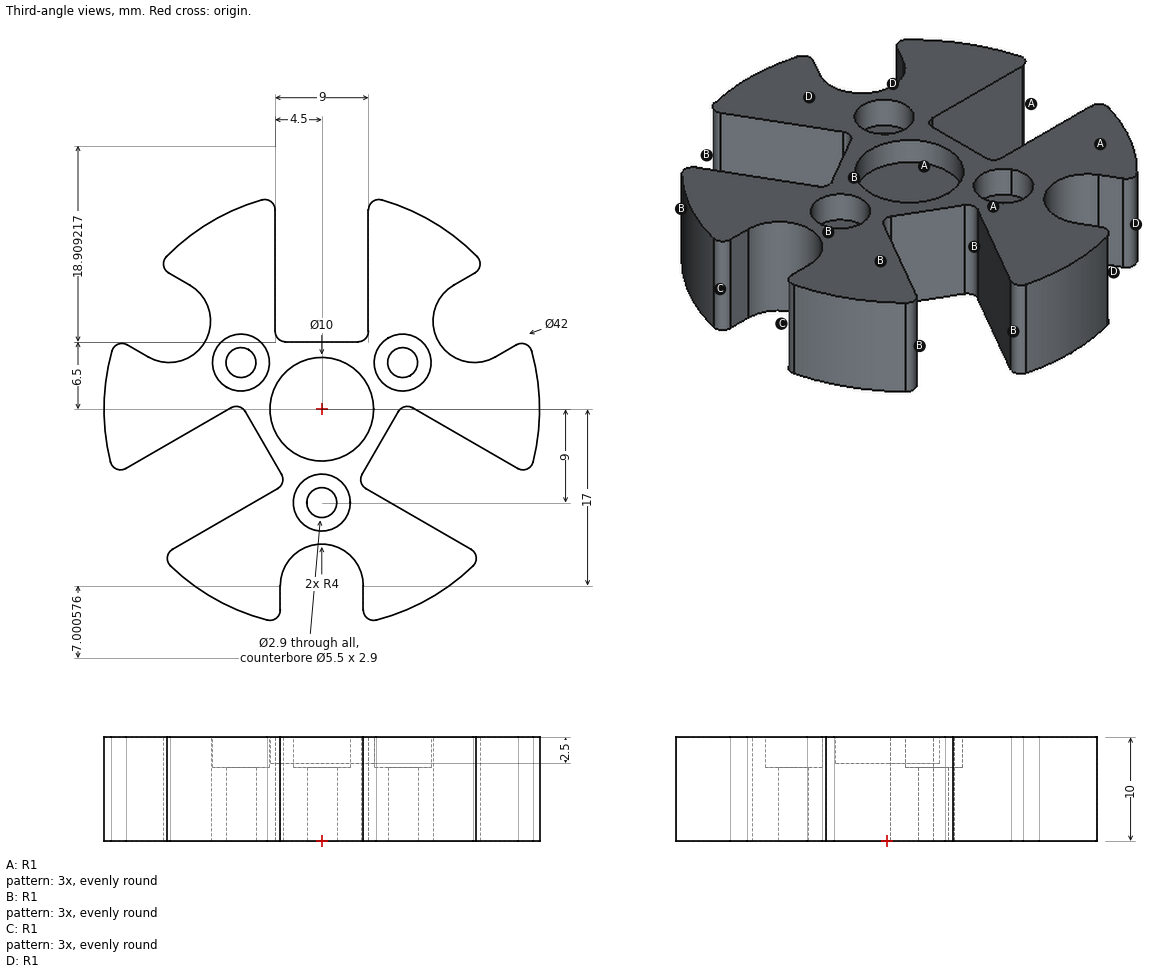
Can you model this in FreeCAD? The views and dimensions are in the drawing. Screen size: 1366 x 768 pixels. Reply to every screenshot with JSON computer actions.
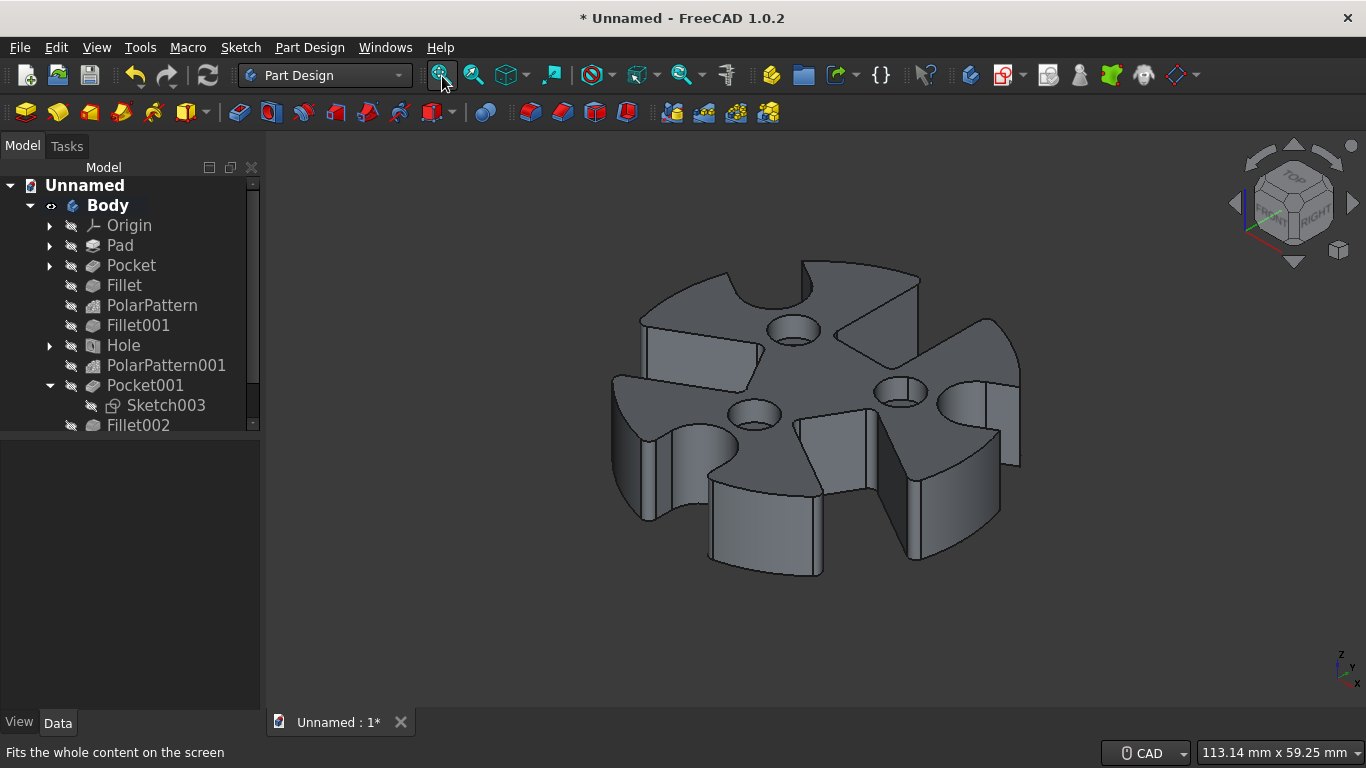
{"action": "left_click", "coordinate": [1020, 426]}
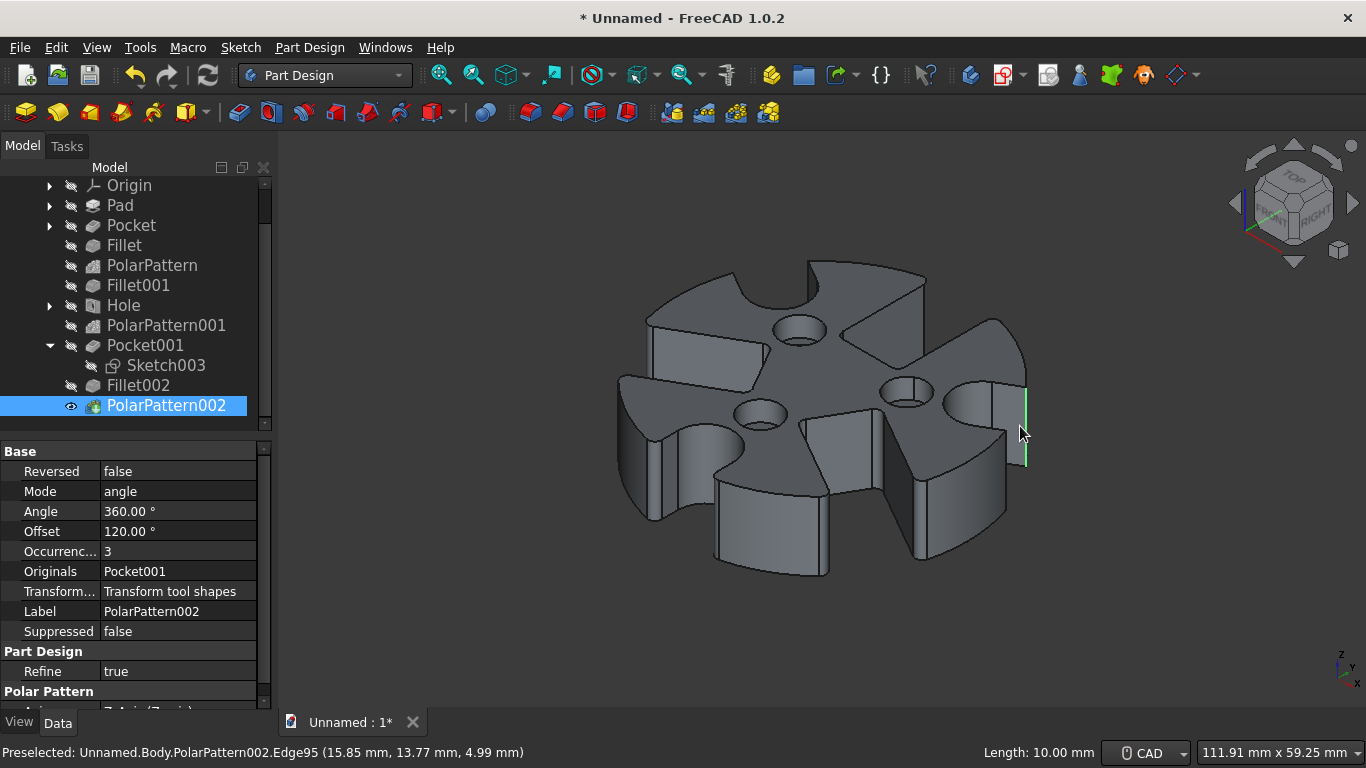
{"action": "key", "text": "2"}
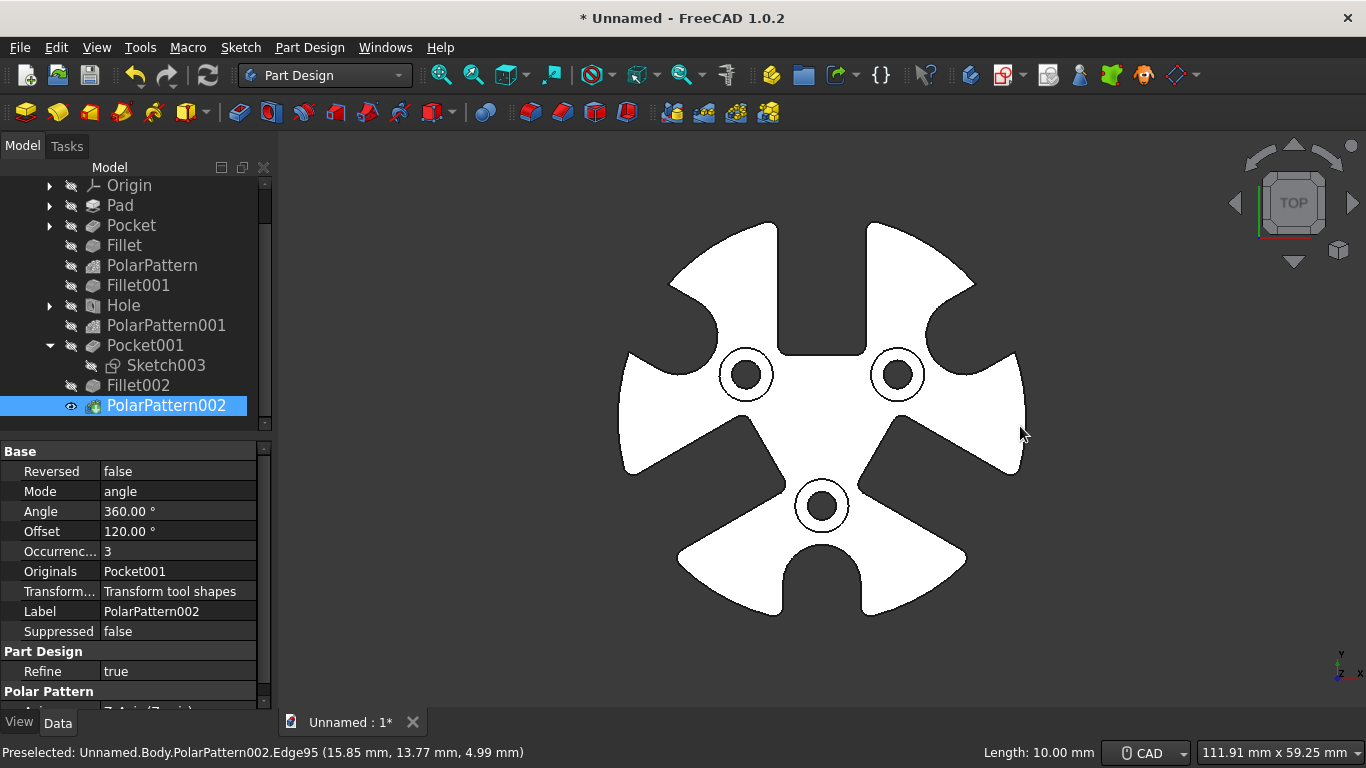
{"action": "key", "text": "1"}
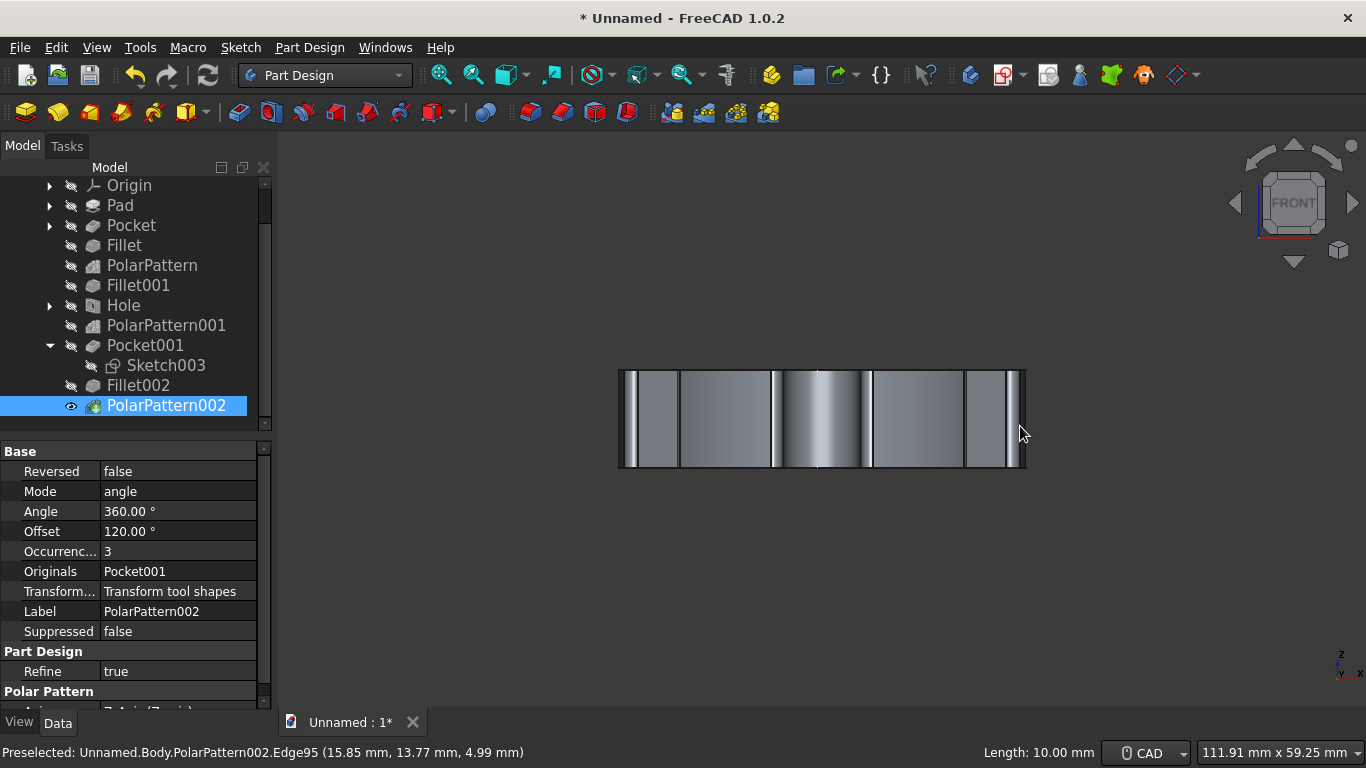
{"action": "left_click", "coordinate": [442, 76]}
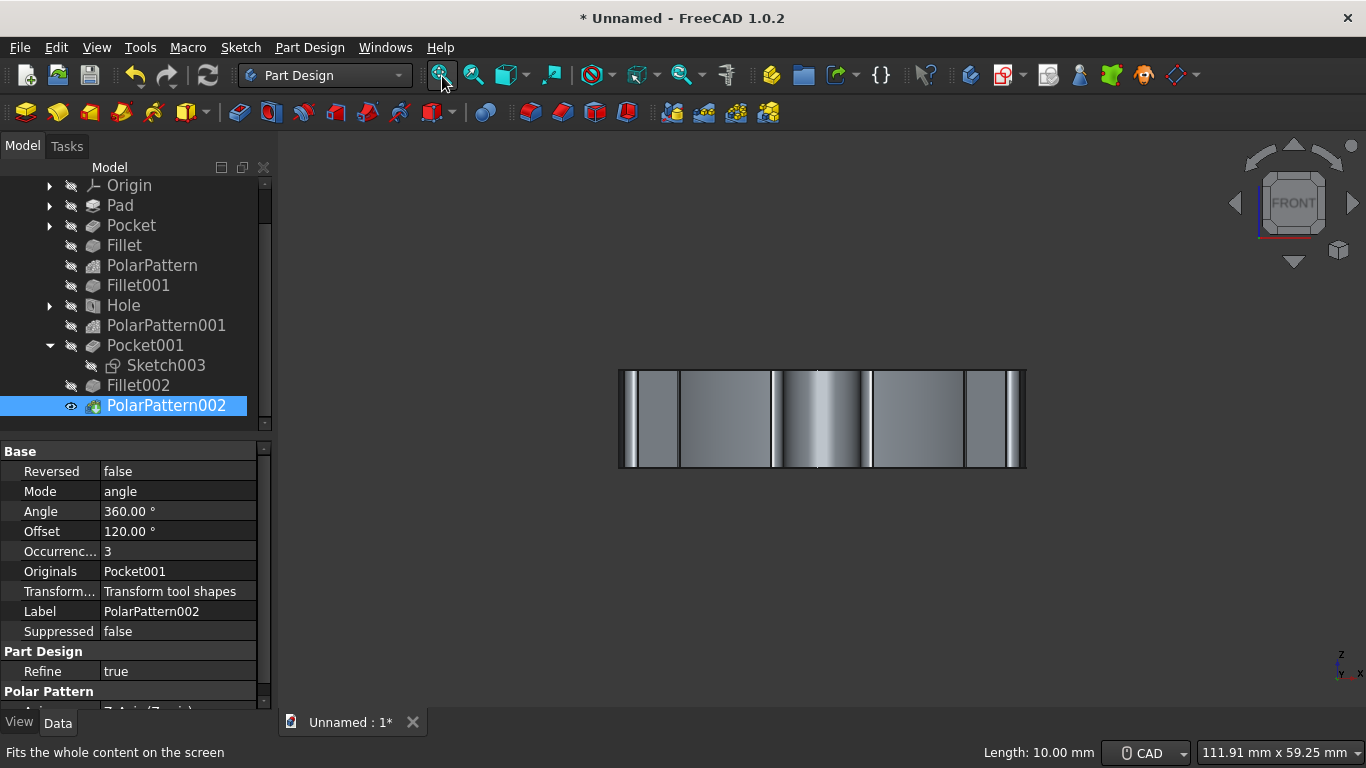
{"action": "key", "text": "3"}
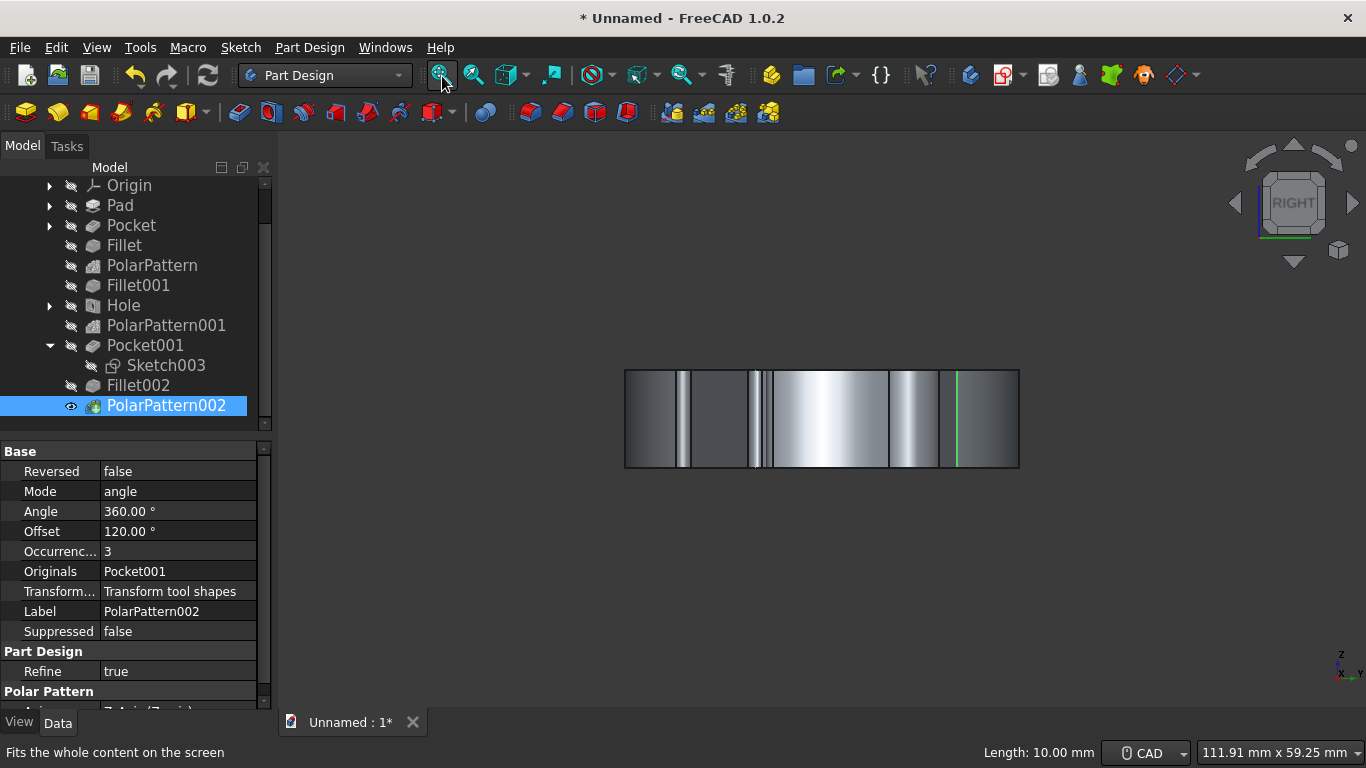
{"action": "left_click", "coordinate": [442, 76]}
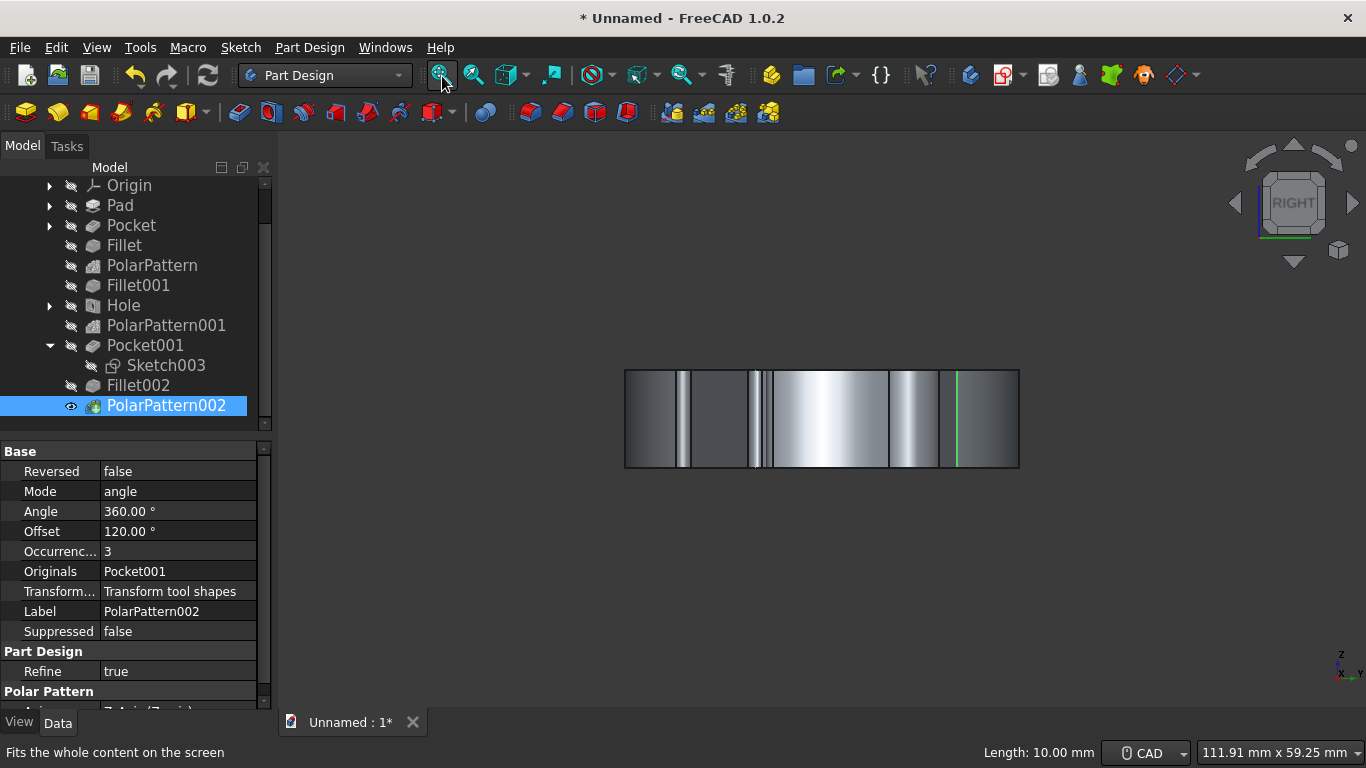
{"action": "key", "text": "5"}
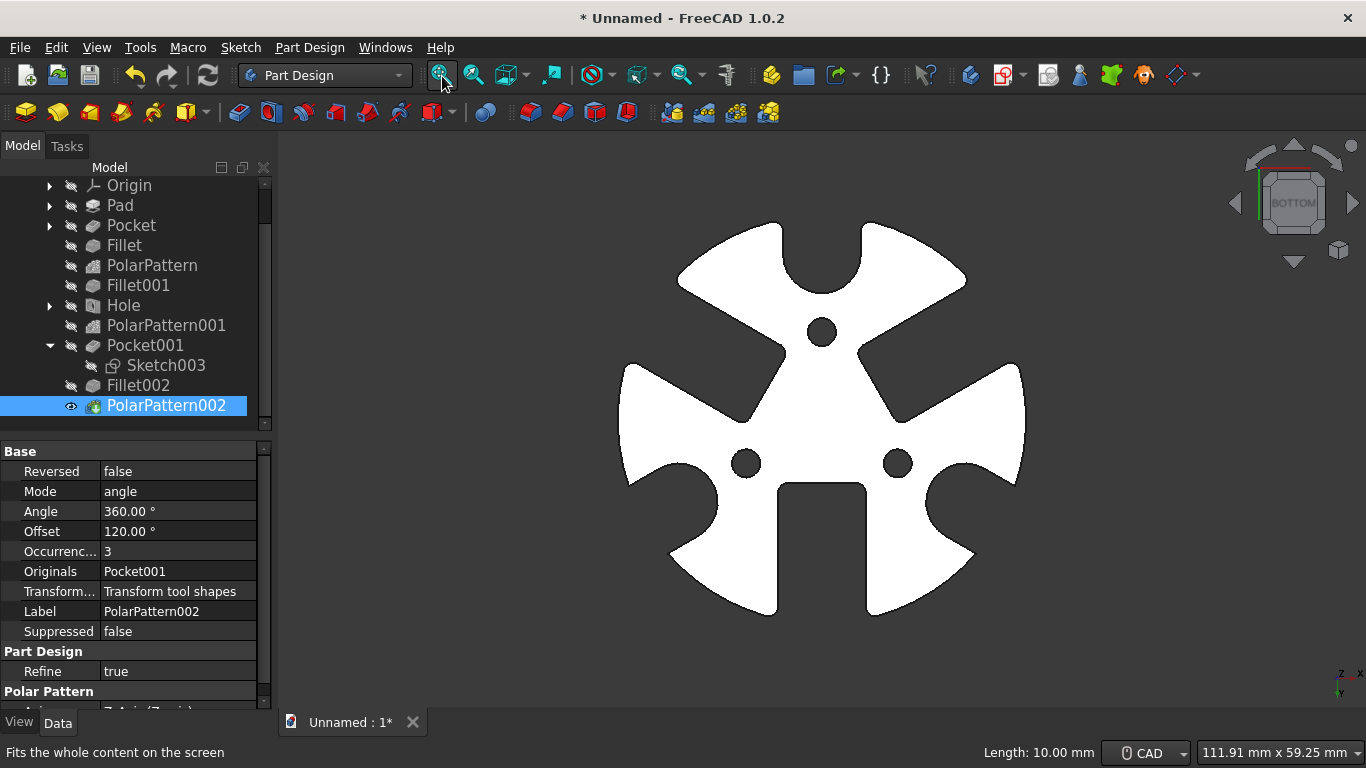
{"action": "key", "text": "4"}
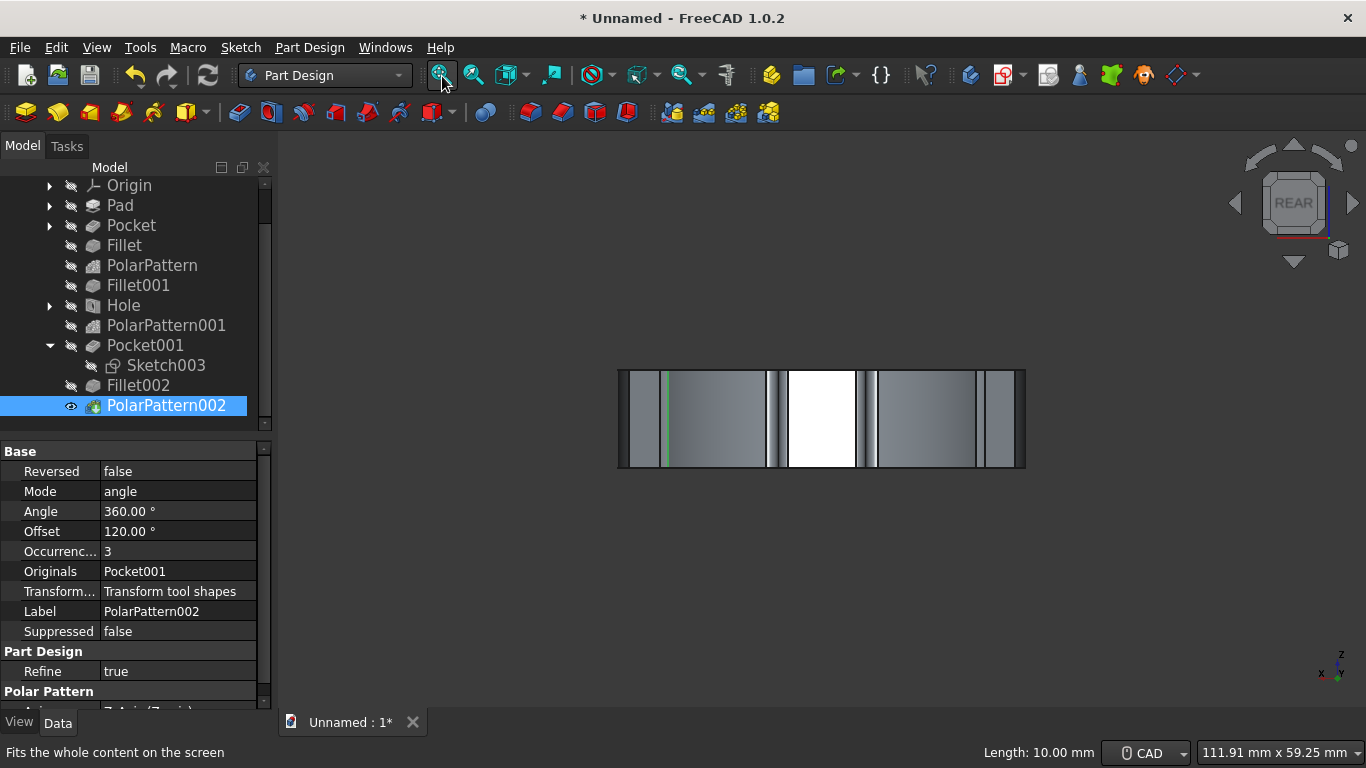
{"action": "left_click", "coordinate": [442, 76]}